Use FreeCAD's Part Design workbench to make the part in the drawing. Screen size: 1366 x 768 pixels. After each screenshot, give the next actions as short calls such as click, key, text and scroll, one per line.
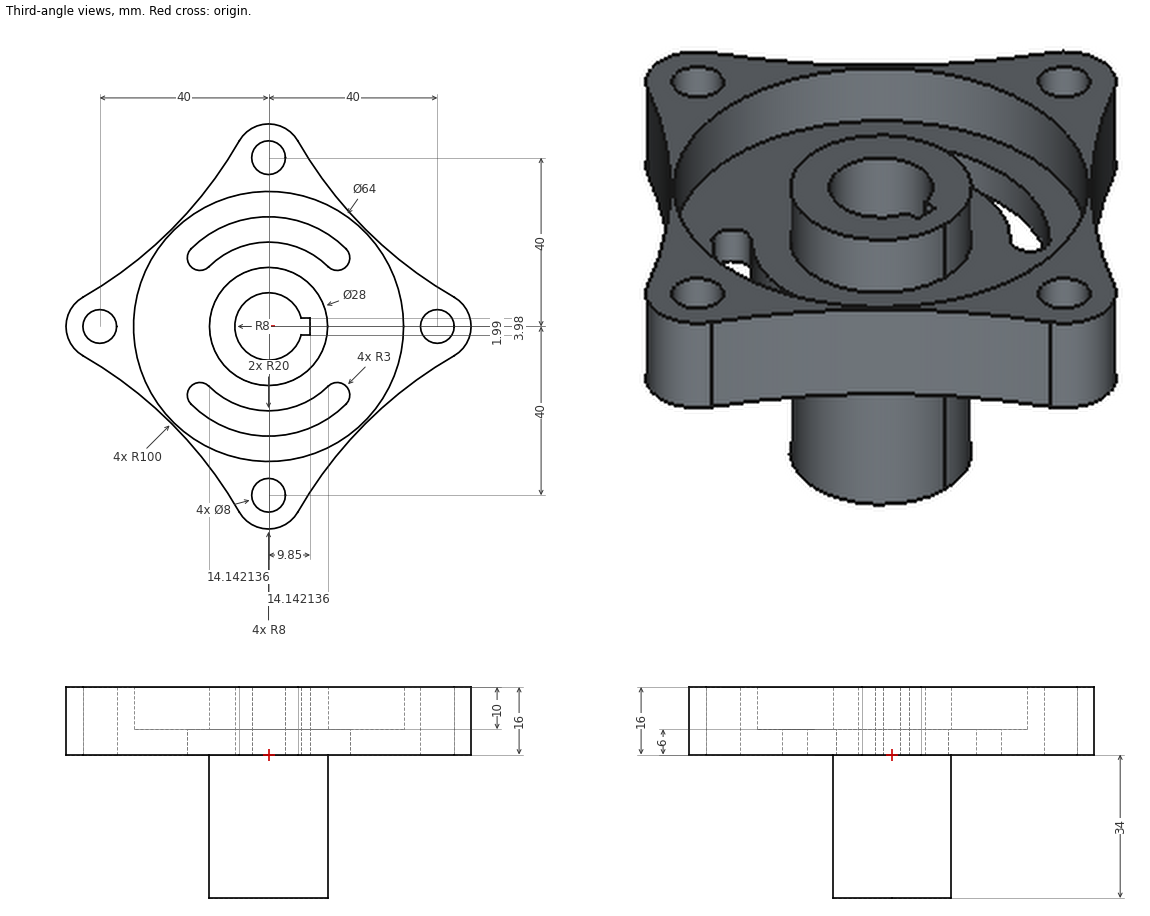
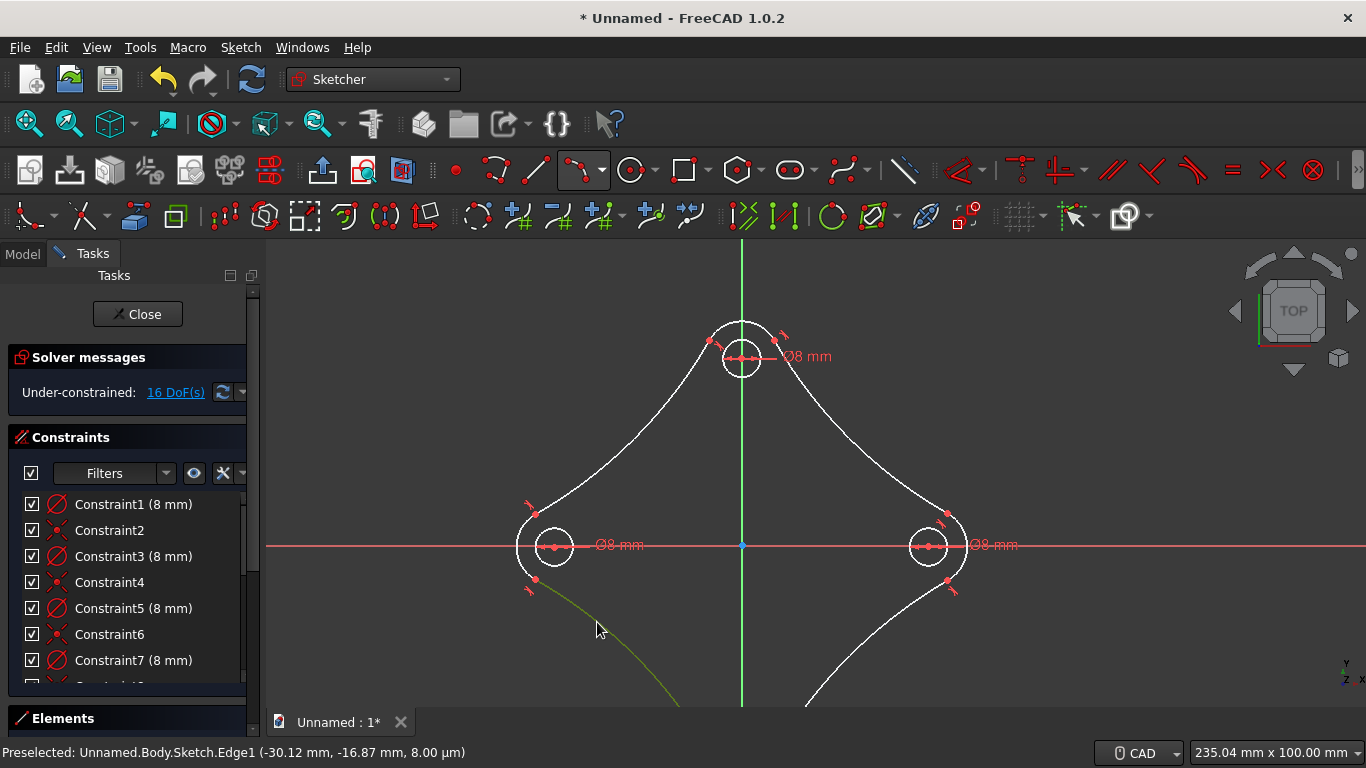
click(887, 623)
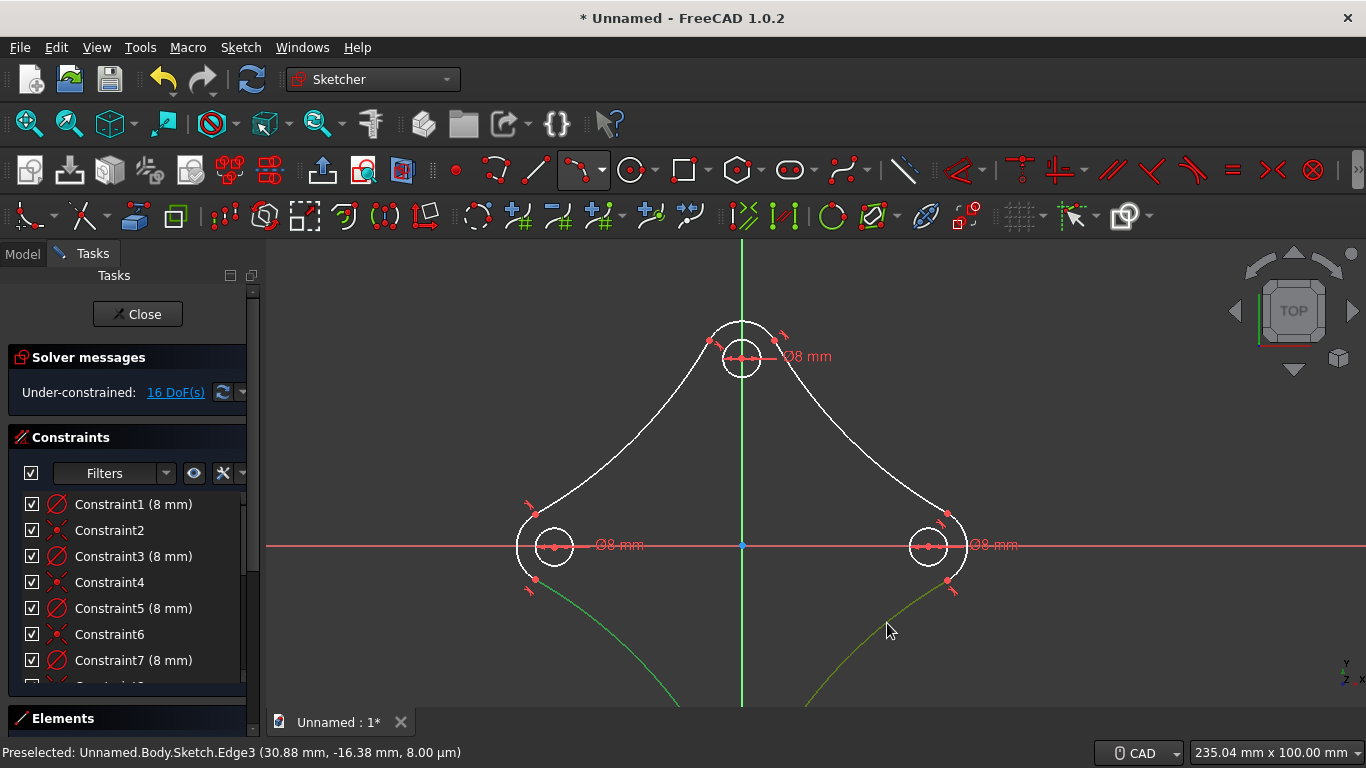
click(816, 402)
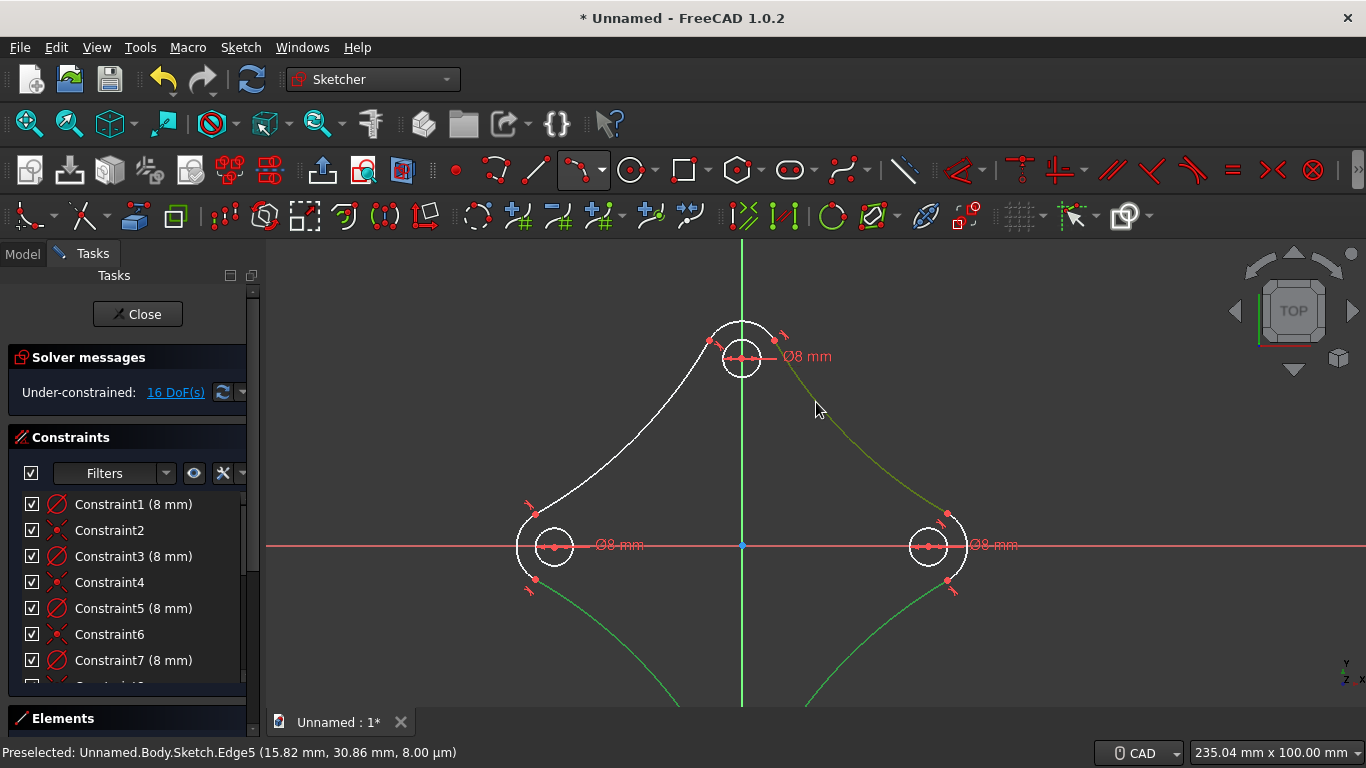
click(597, 472)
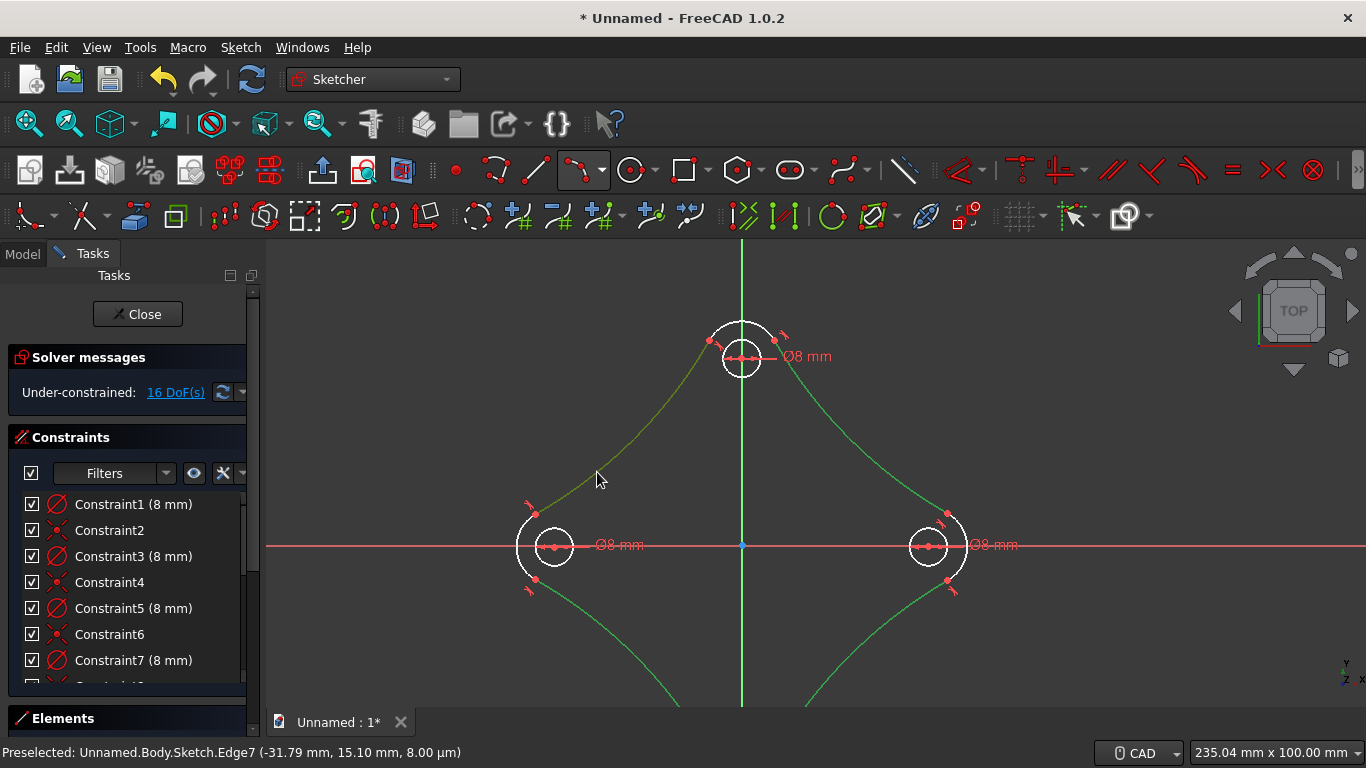
click(1234, 170)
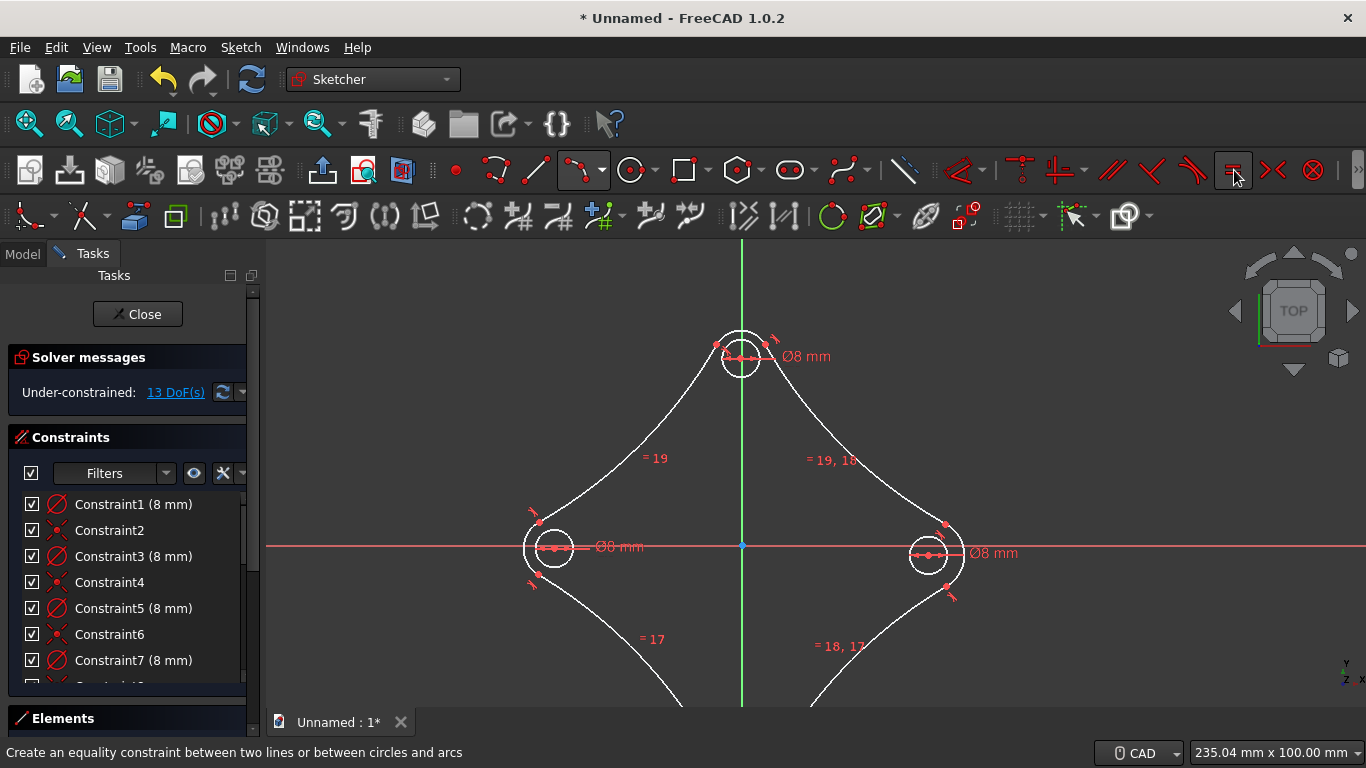
scroll(758, 325, down, 2)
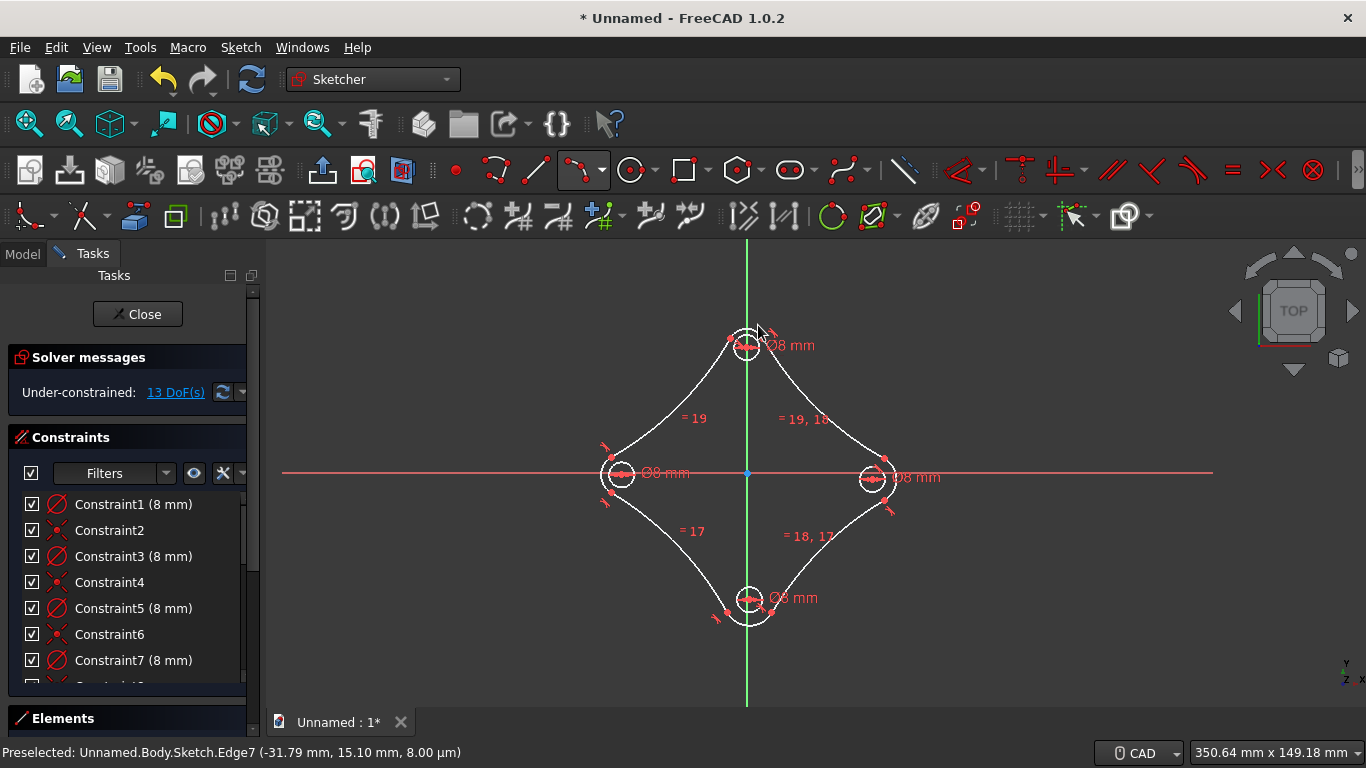
scroll(739, 623, up, 3)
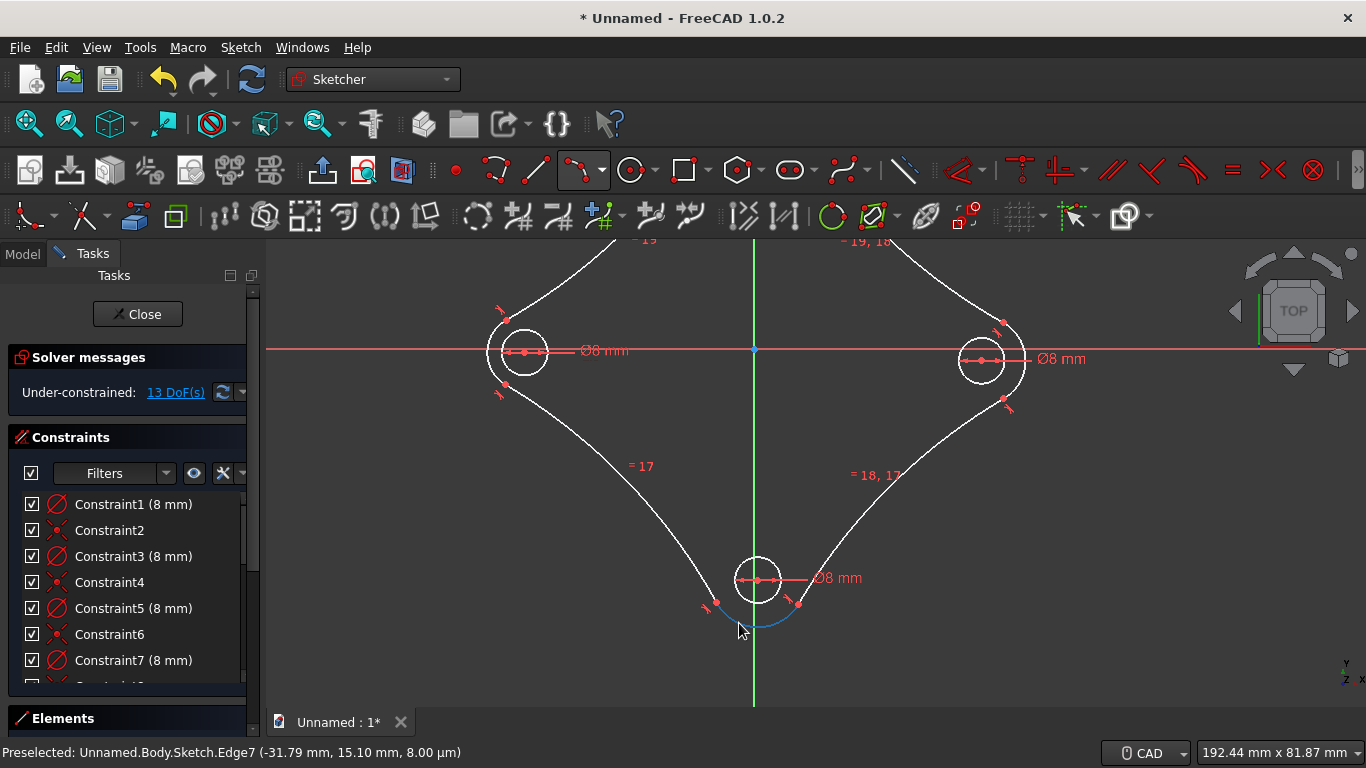
click(738, 623)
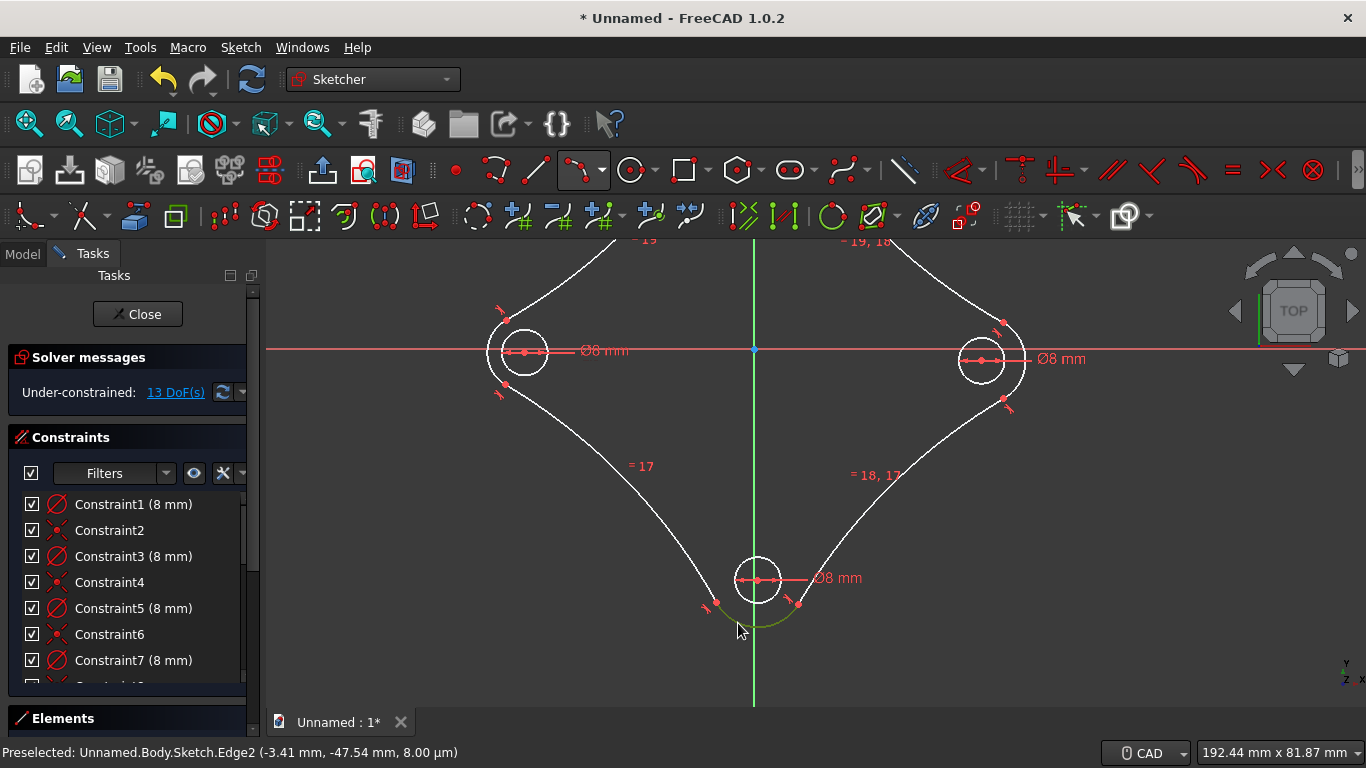
click(1022, 378)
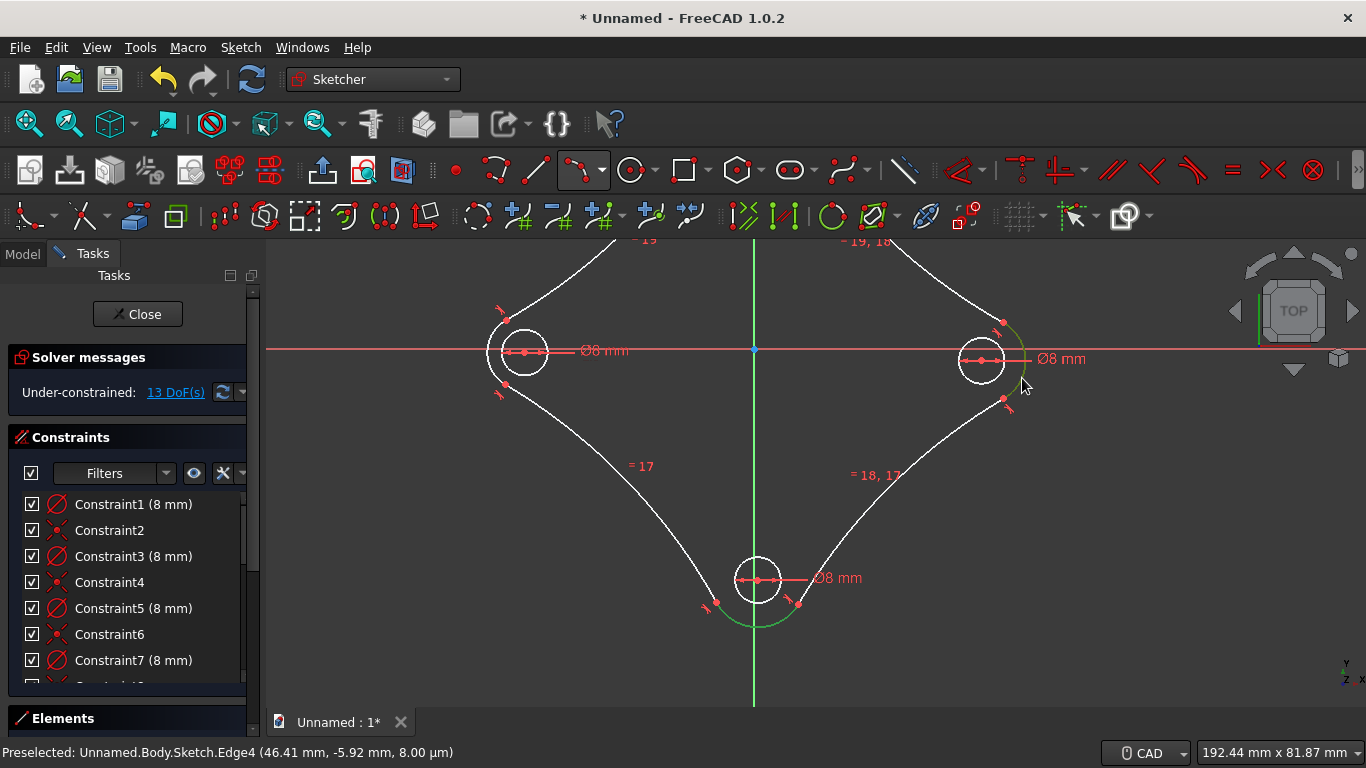
scroll(739, 623, down, 3)